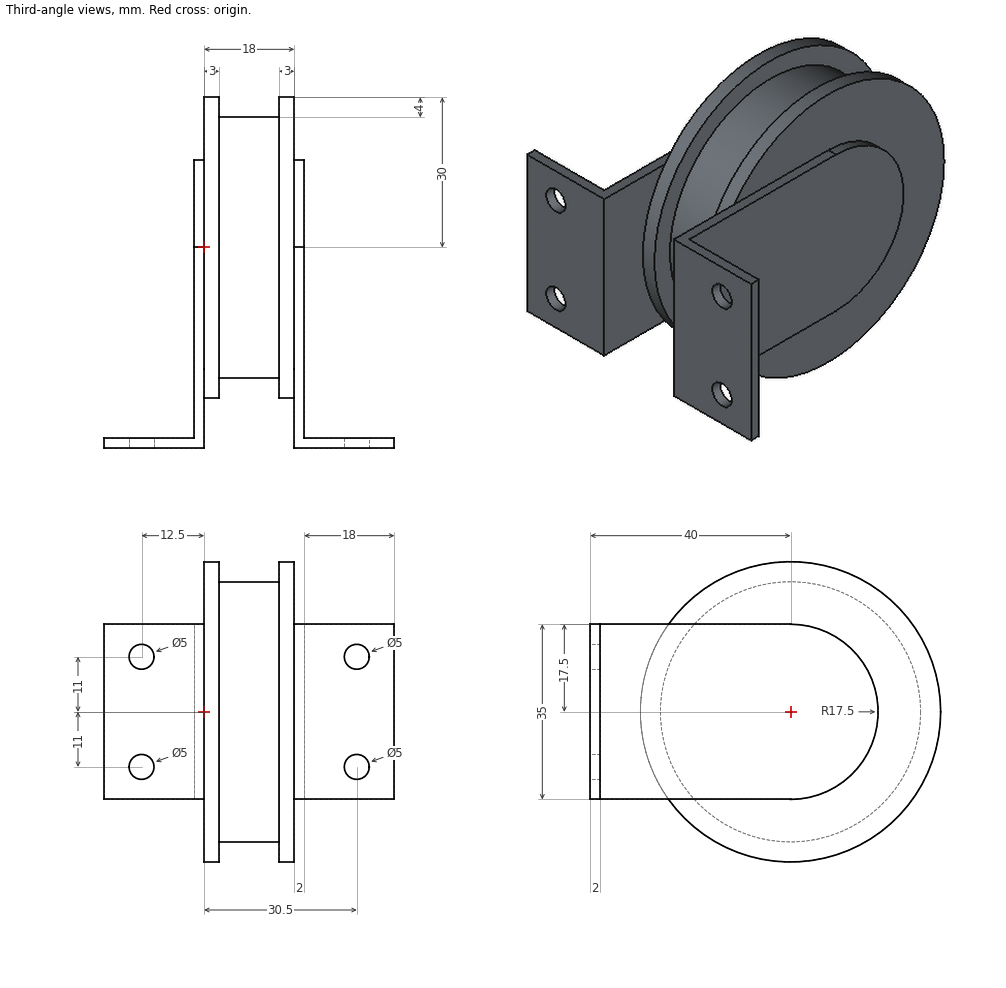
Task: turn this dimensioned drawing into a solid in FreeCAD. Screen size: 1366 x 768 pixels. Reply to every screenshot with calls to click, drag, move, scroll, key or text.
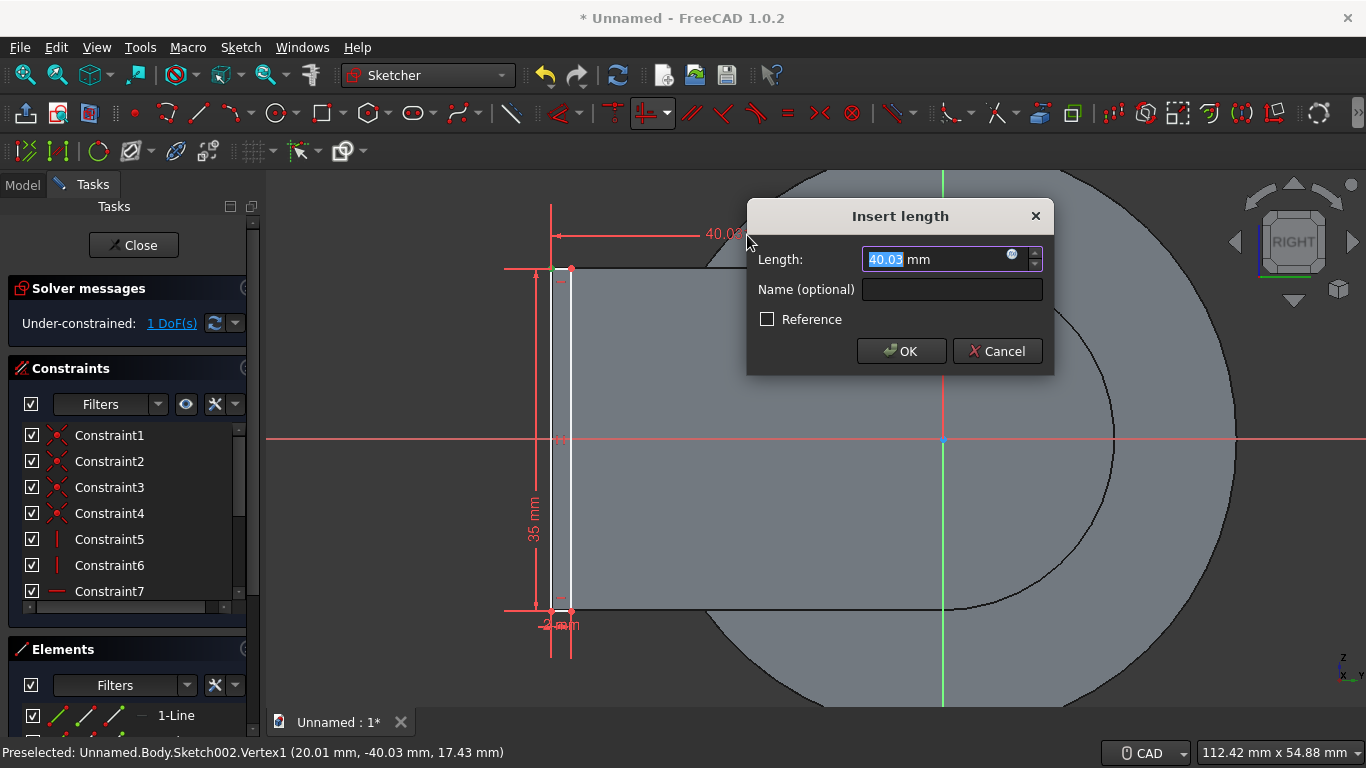
text(40)
key(Return)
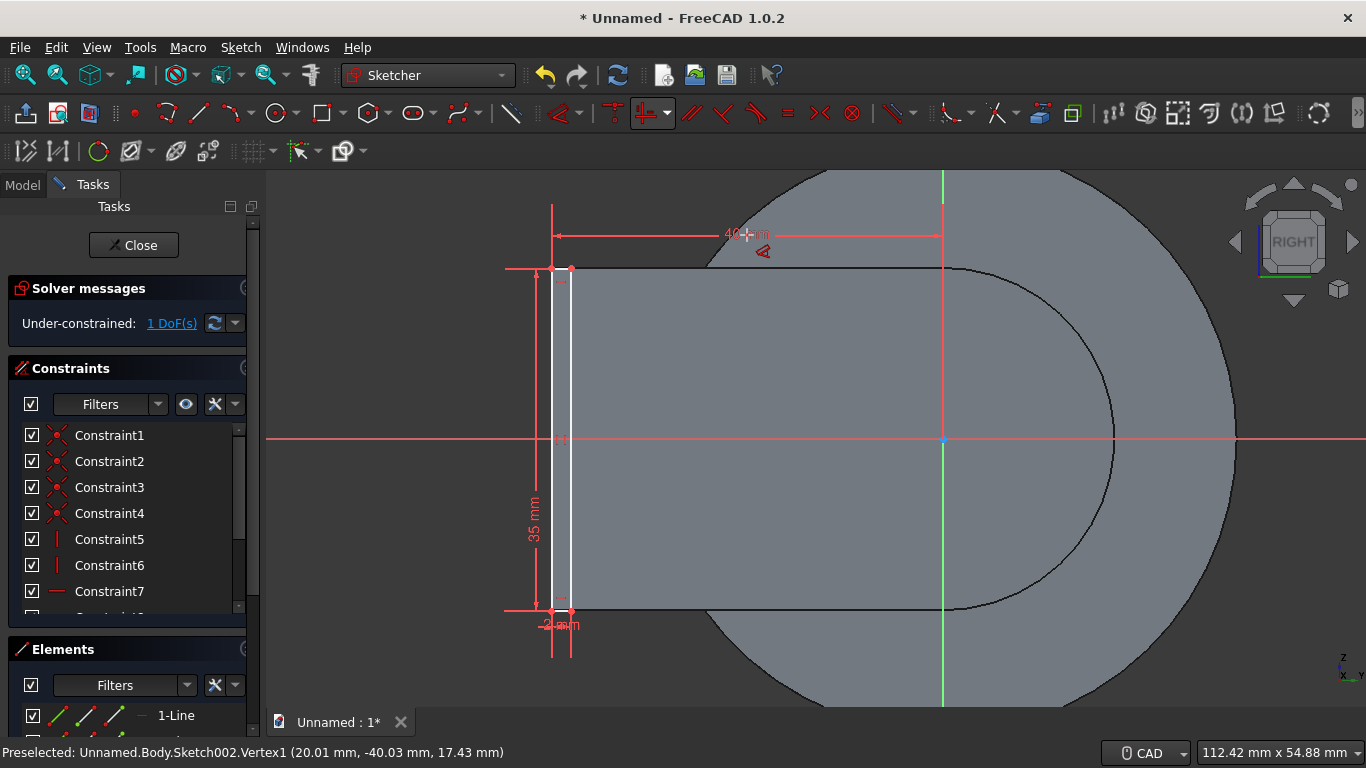
click(552, 269)
click(977, 354)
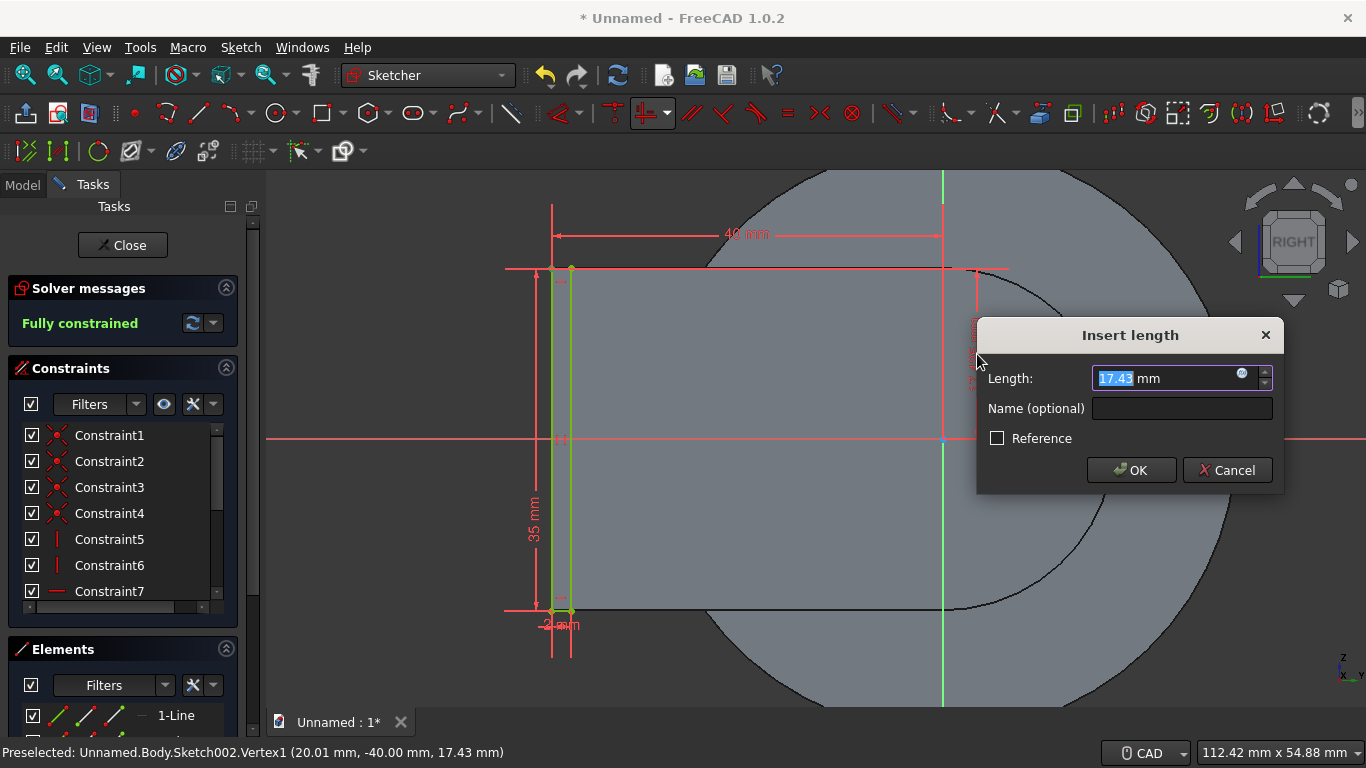
text(17.5)
key(Return)
key(Escape)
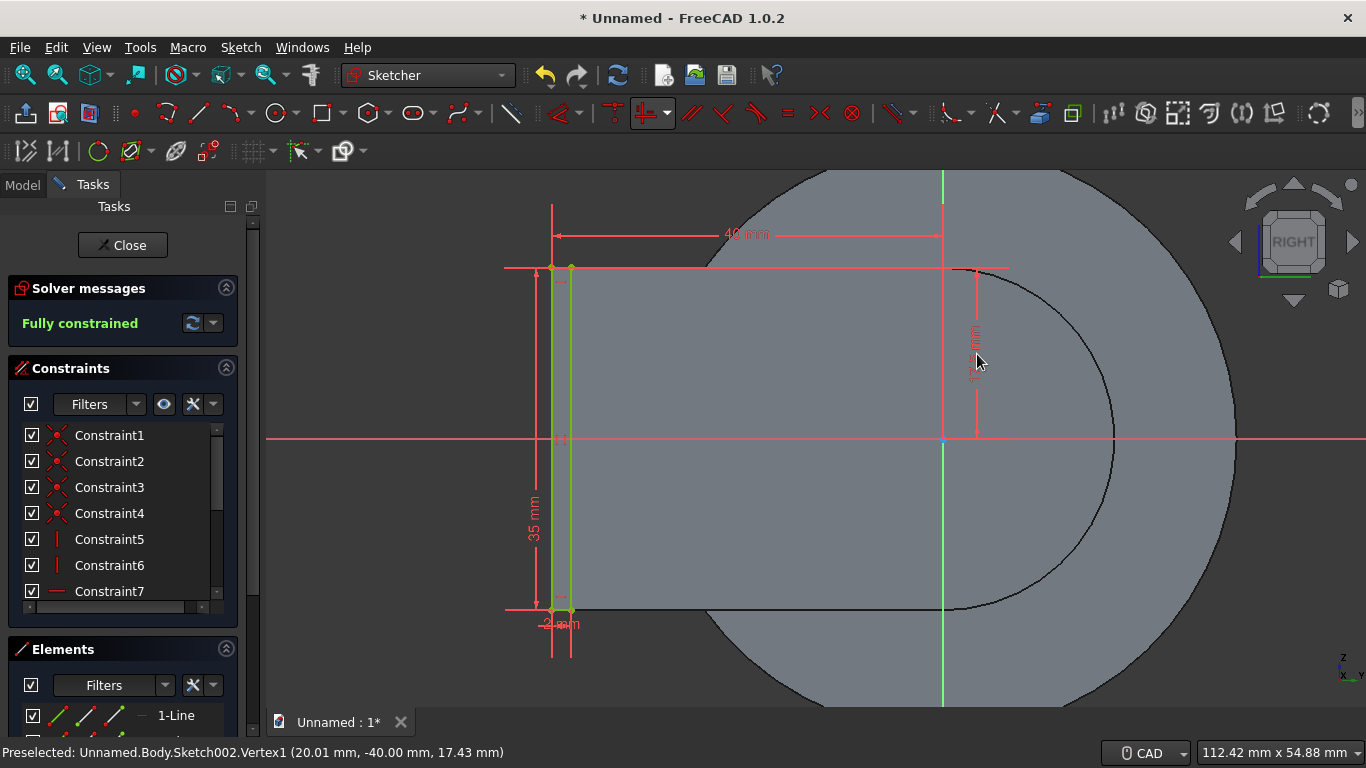
click(123, 245)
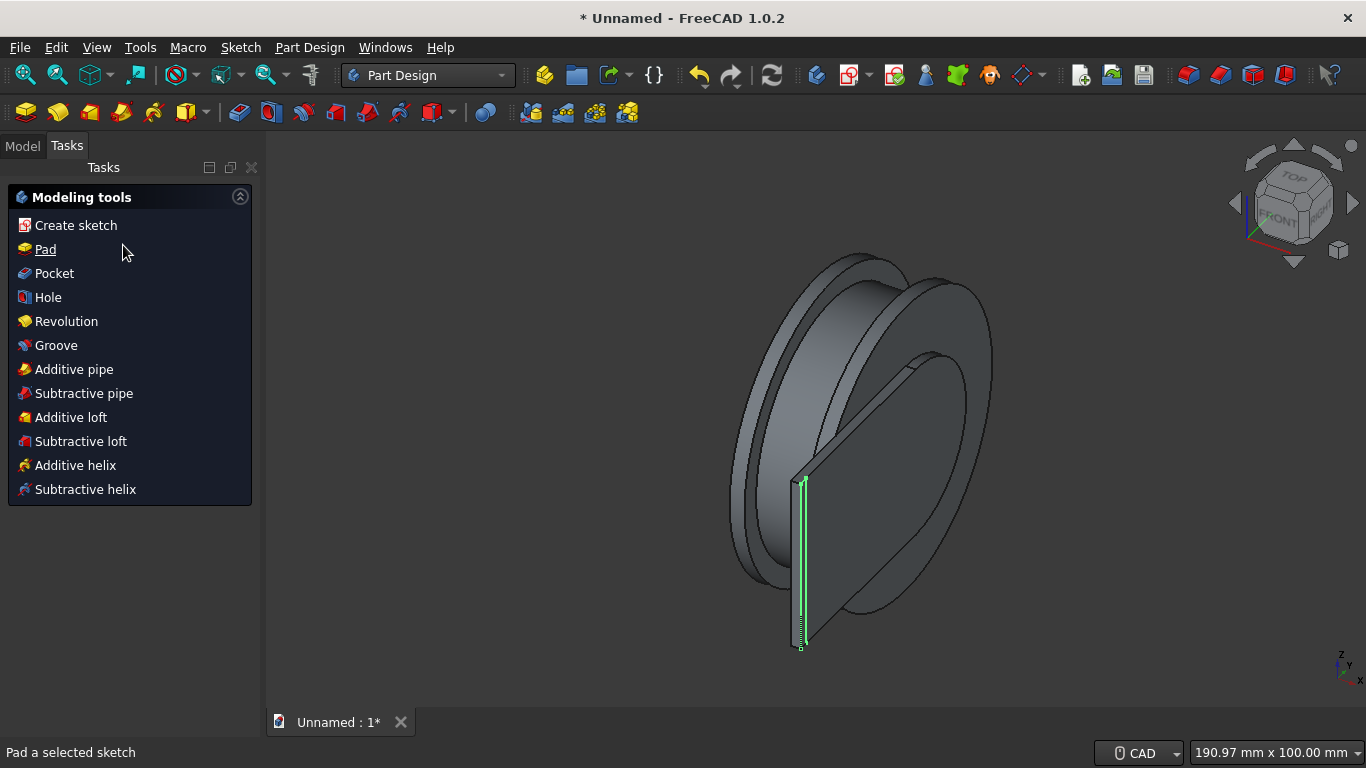
click(26, 112)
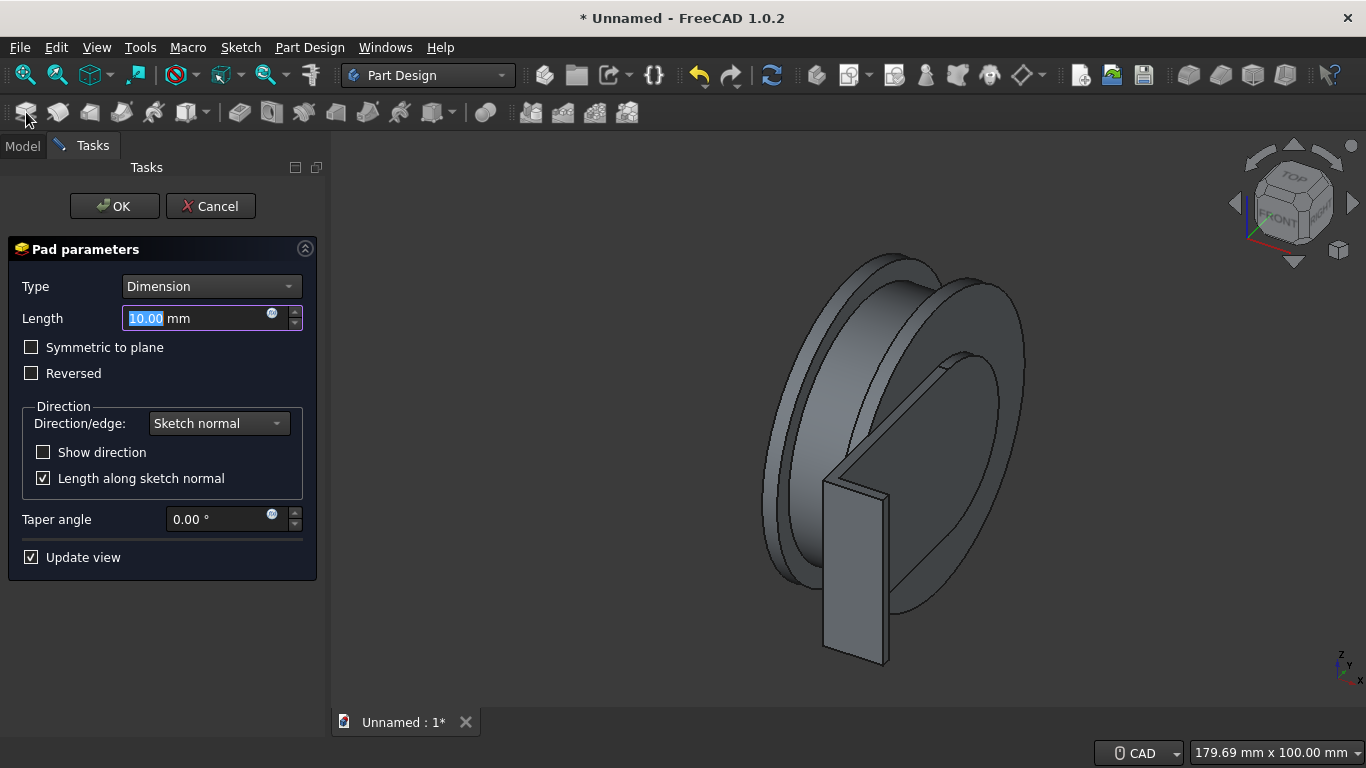
text(18)
key(Tab)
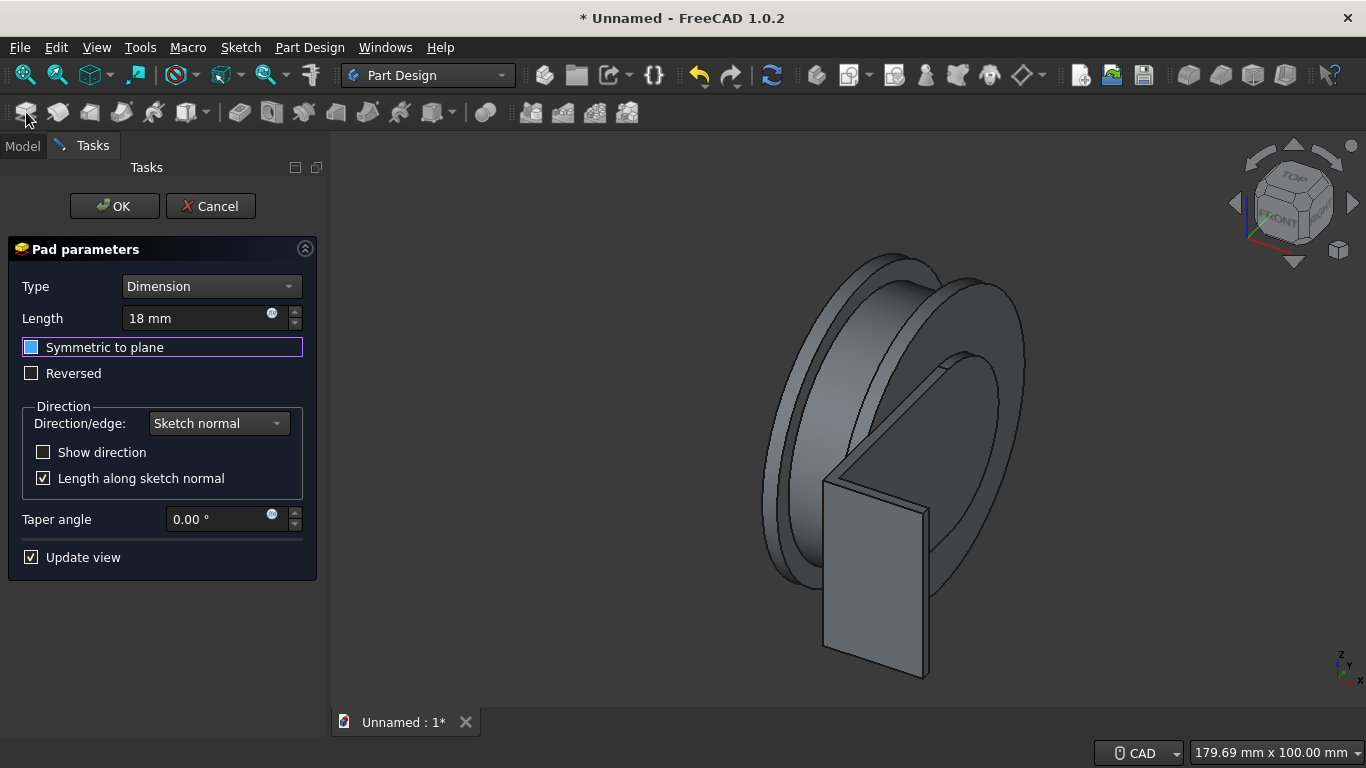
click(115, 206)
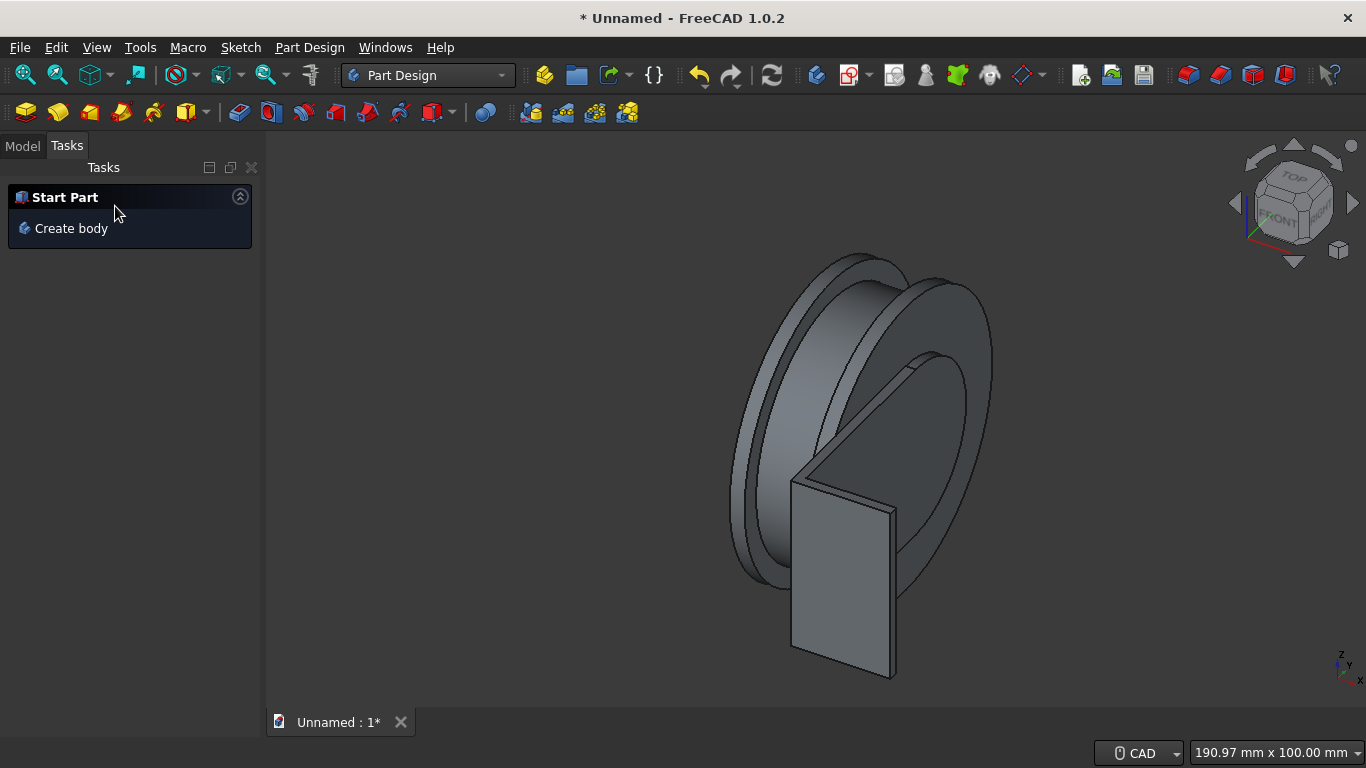
click(26, 76)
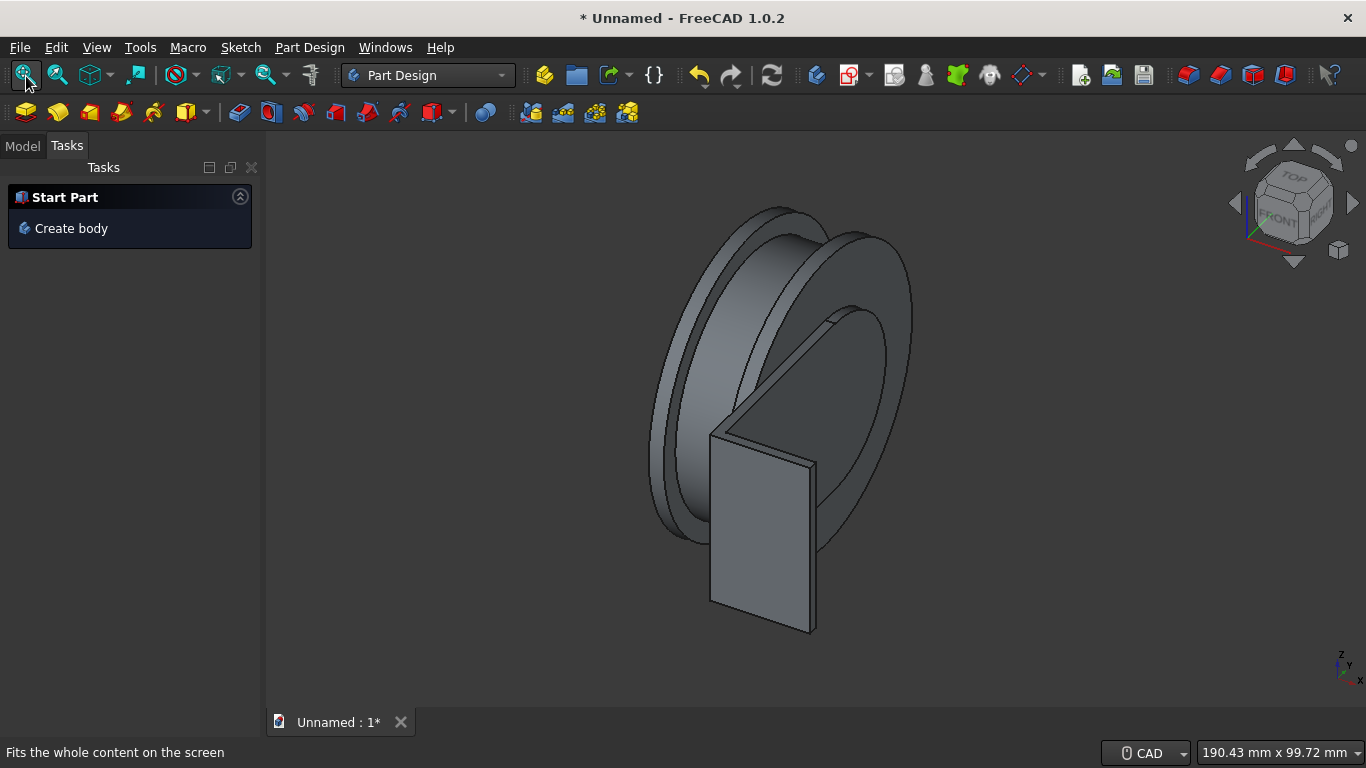
click(23, 145)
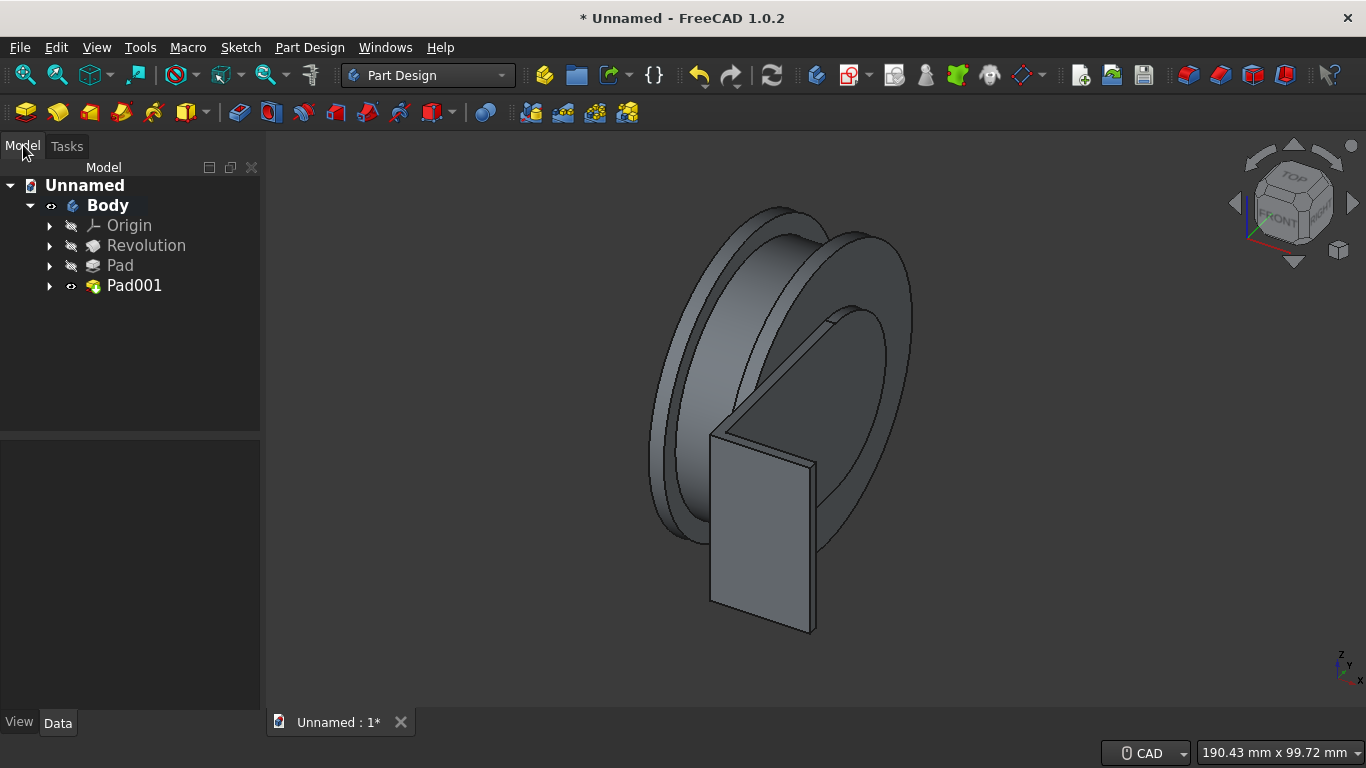
click(50, 226)